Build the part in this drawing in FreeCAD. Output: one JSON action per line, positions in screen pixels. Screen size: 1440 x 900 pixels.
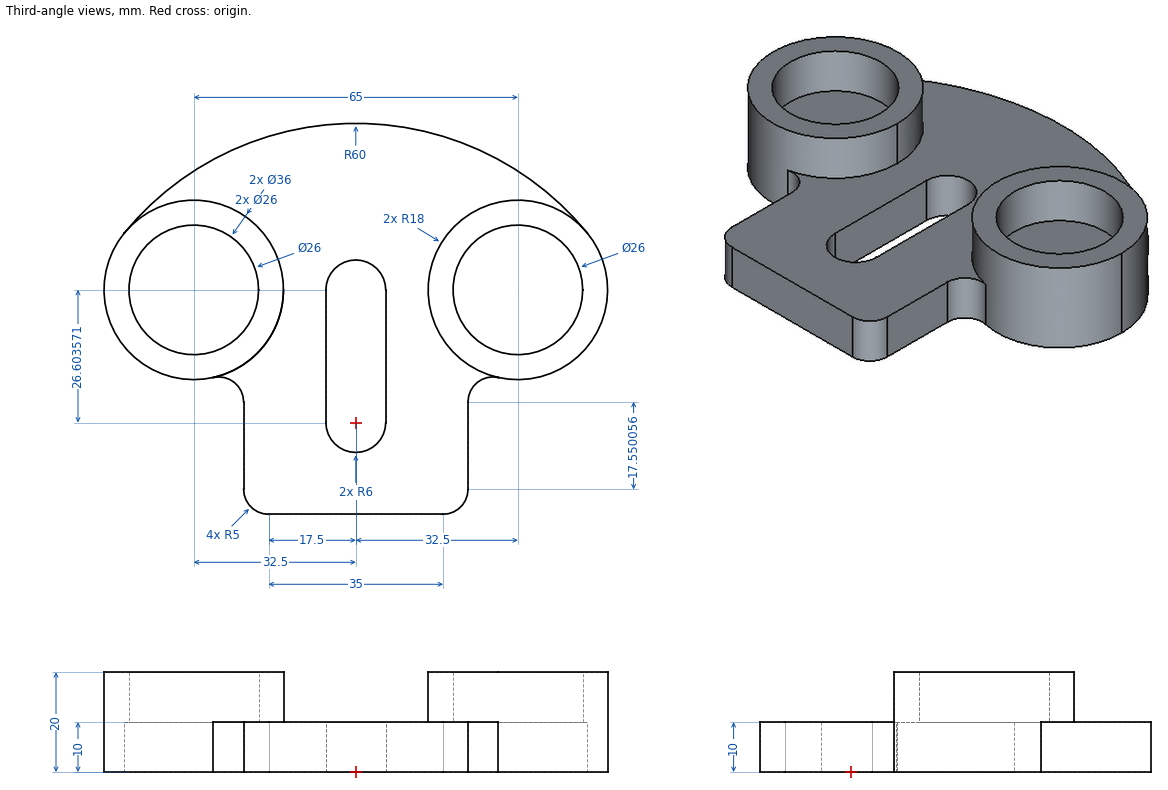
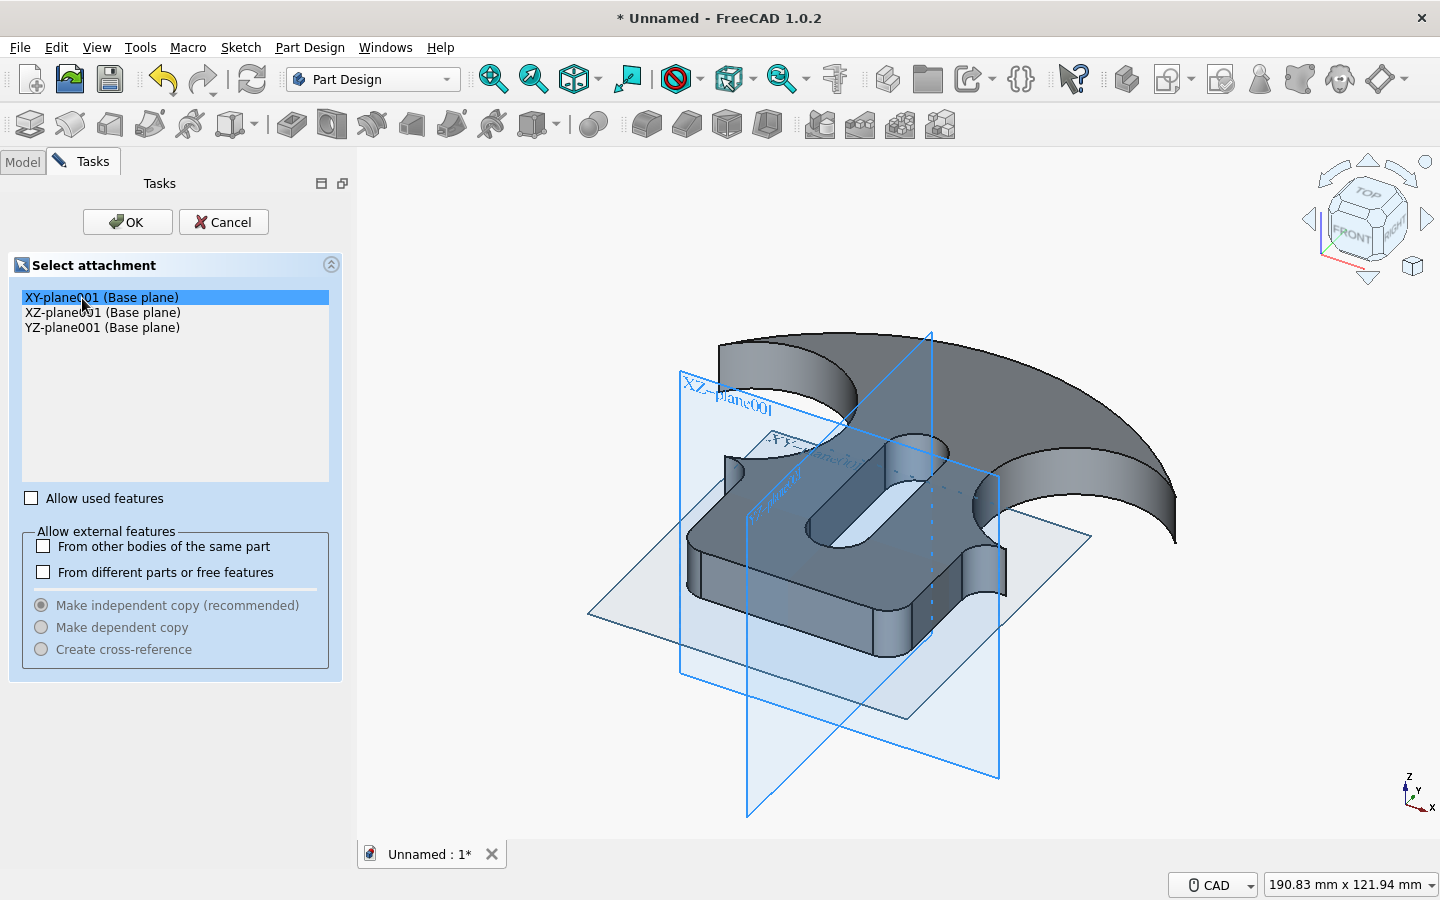
{"action": "left_click", "coordinate": [128, 222]}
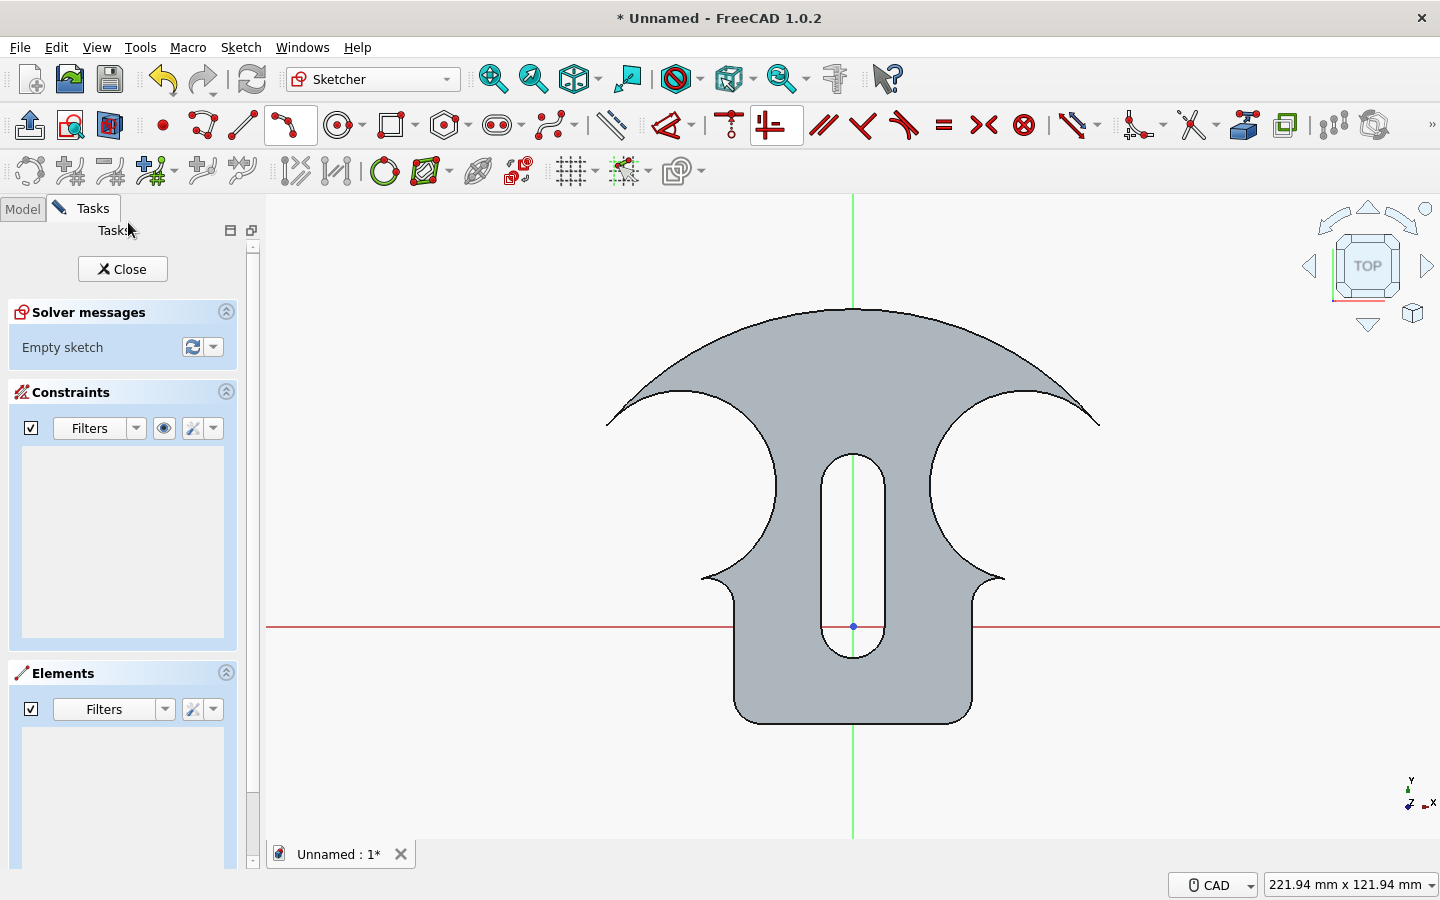
{"action": "scroll", "coordinate": [670, 528], "scroll_direction": "up", "scroll_amount": 3}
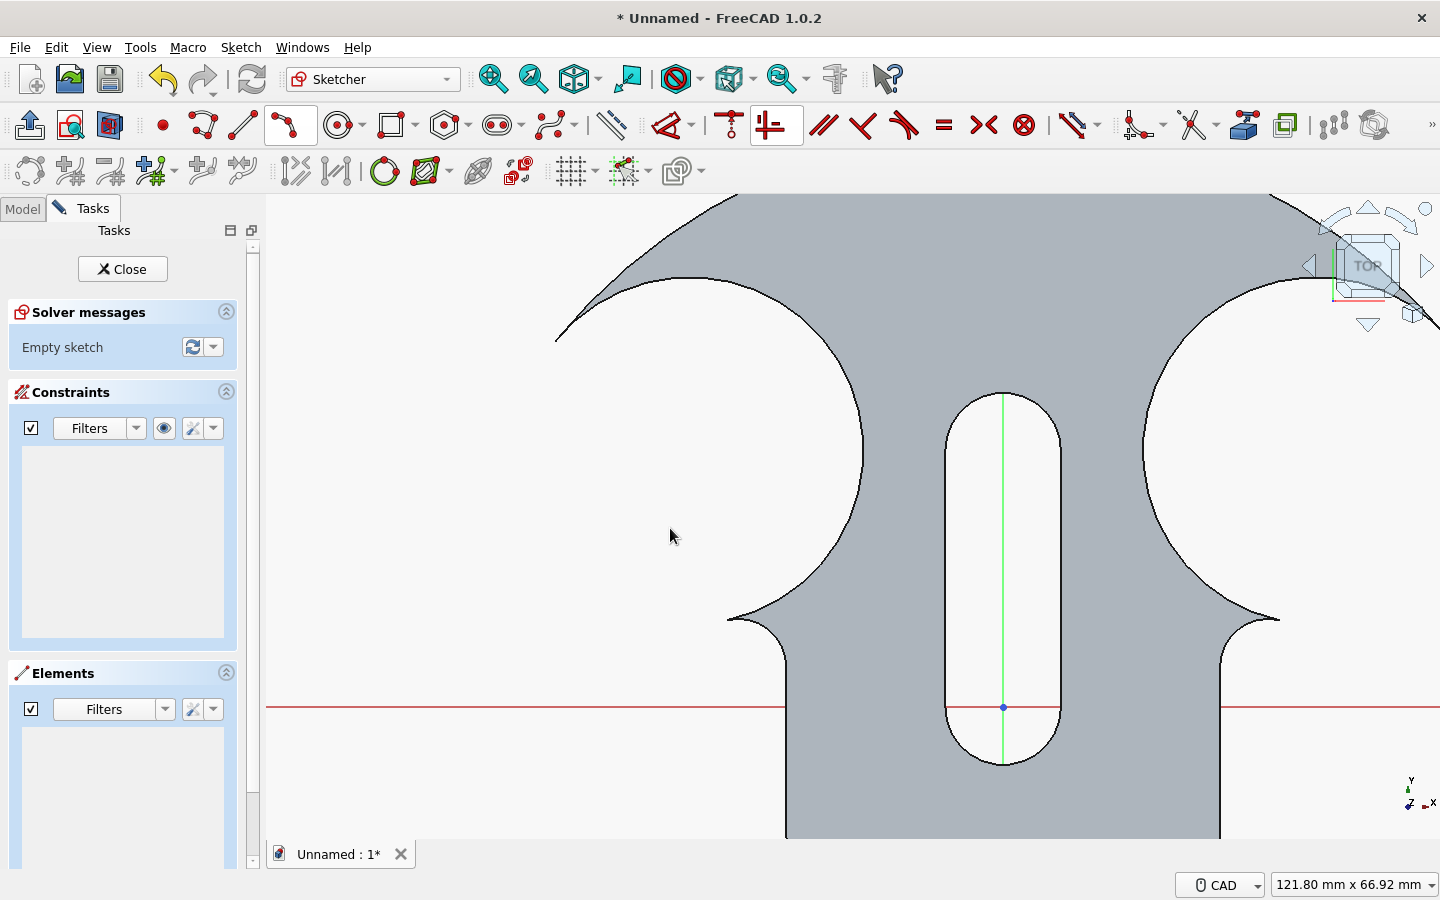
{"action": "left_click", "coordinate": [338, 126]}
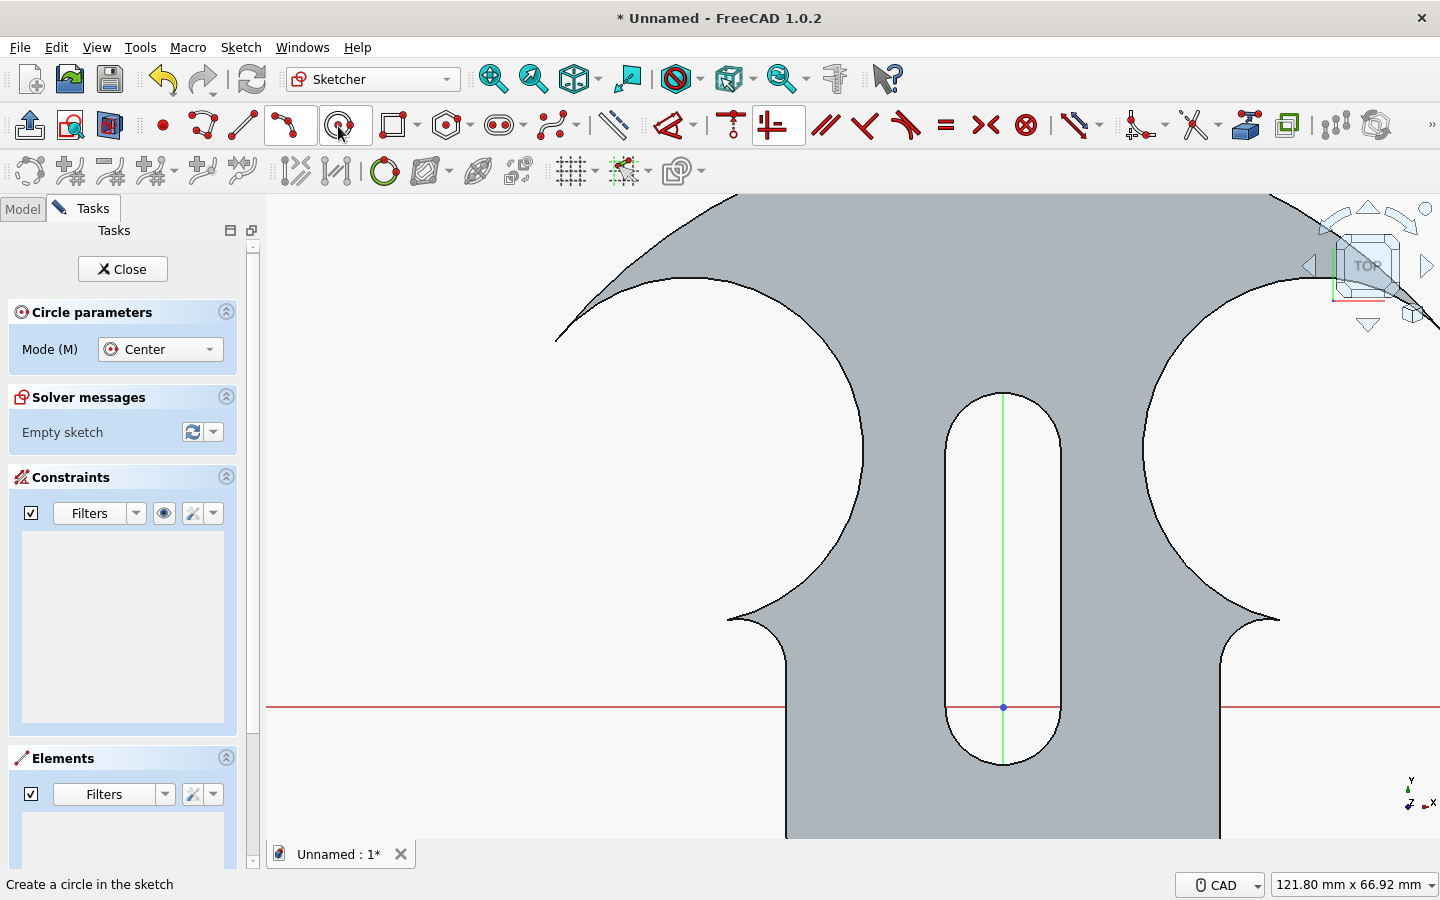
{"action": "left_click", "coordinate": [690, 451]}
{"action": "mouse_move", "coordinate": [779, 362]}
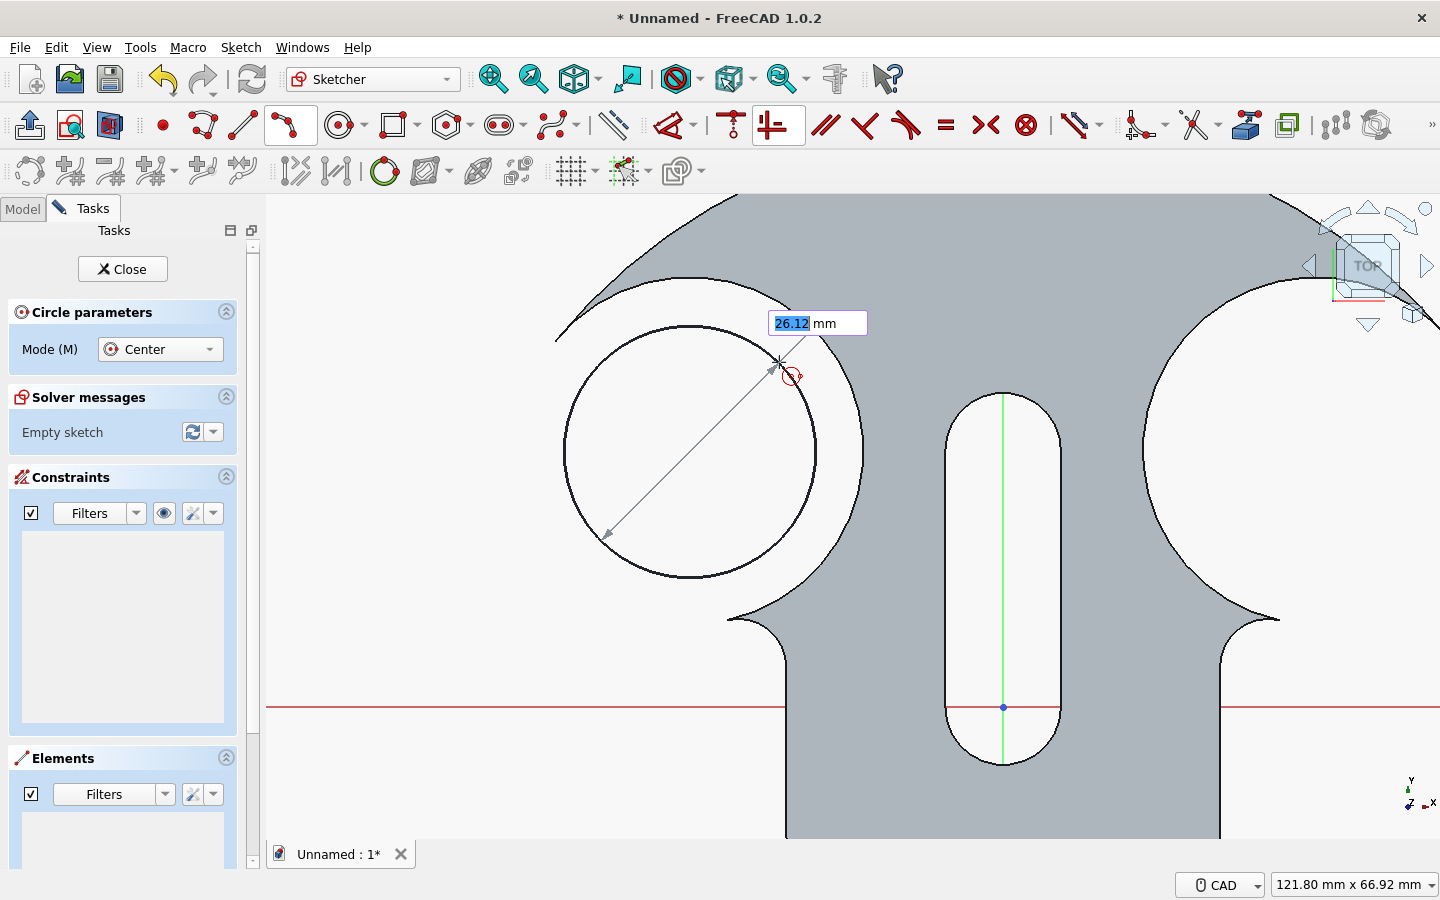
{"action": "type", "text": "26"}
{"action": "key", "text": "Return"}
{"action": "key", "text": "Escape"}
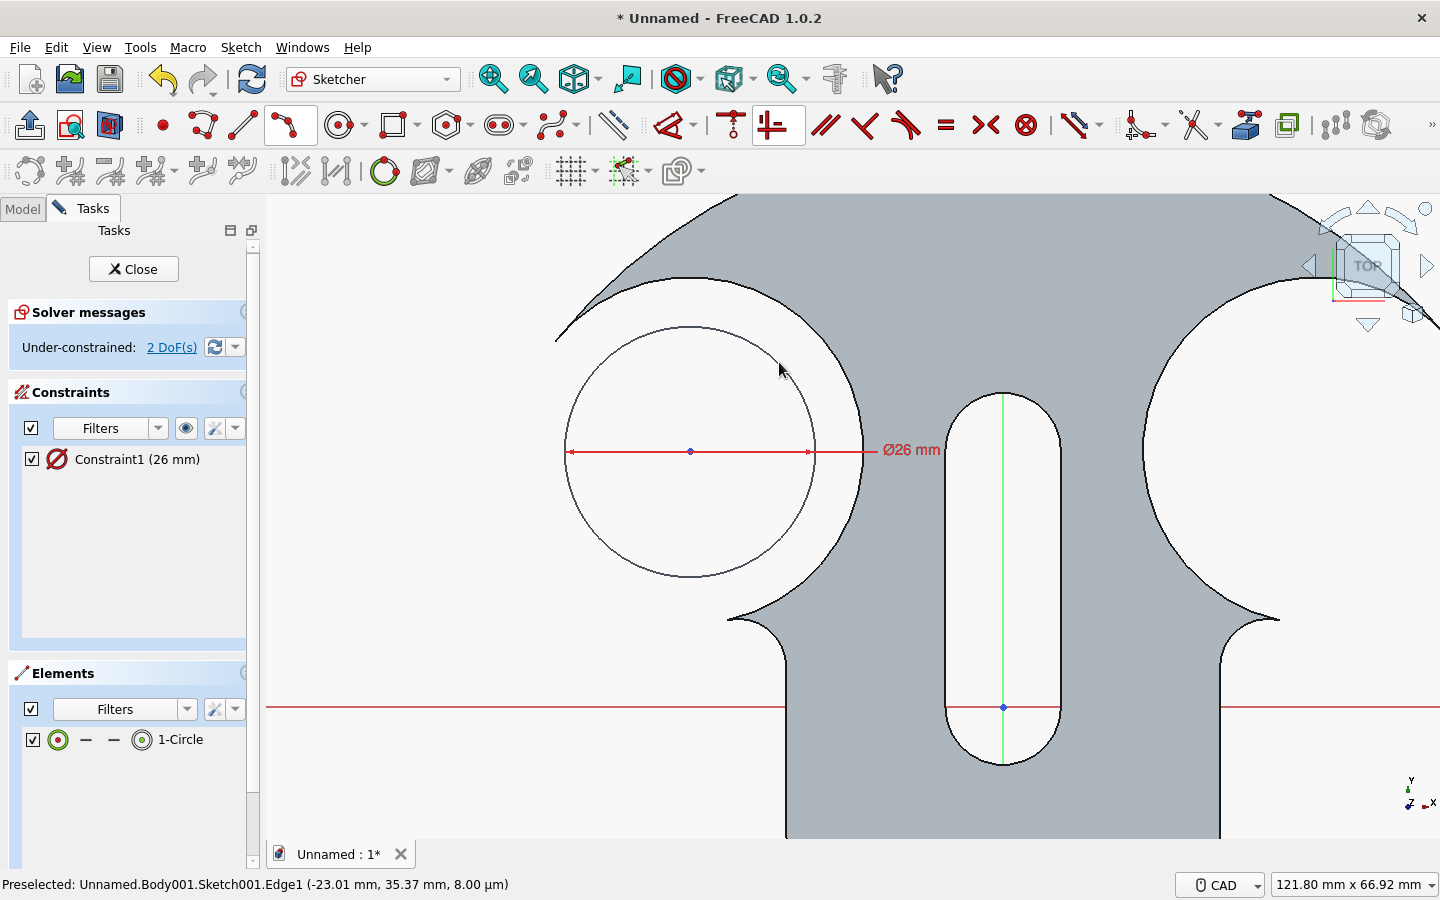
{"action": "left_click", "coordinate": [668, 126]}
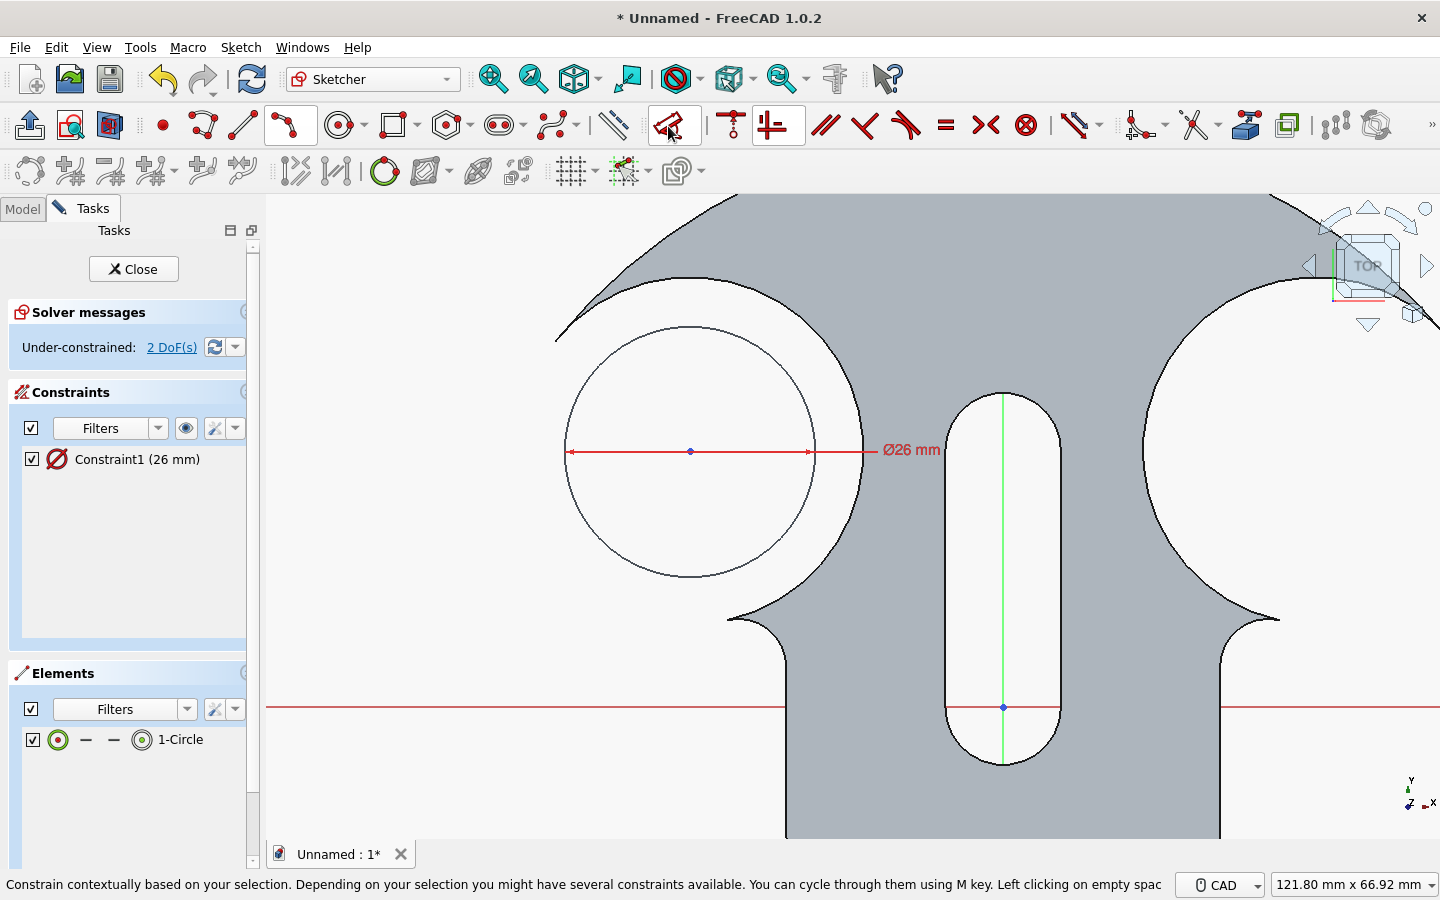
{"action": "left_click", "coordinate": [690, 452]}
{"action": "left_click", "coordinate": [847, 741]}